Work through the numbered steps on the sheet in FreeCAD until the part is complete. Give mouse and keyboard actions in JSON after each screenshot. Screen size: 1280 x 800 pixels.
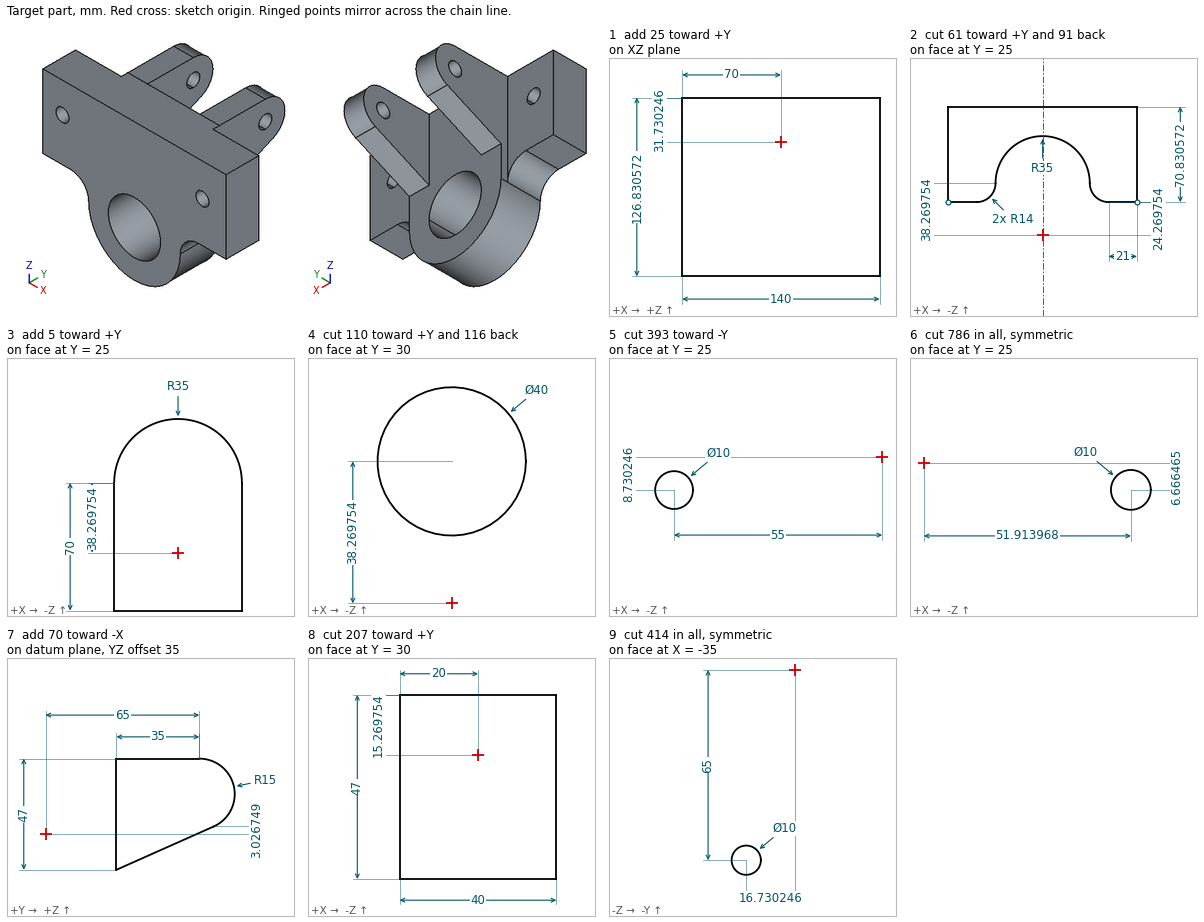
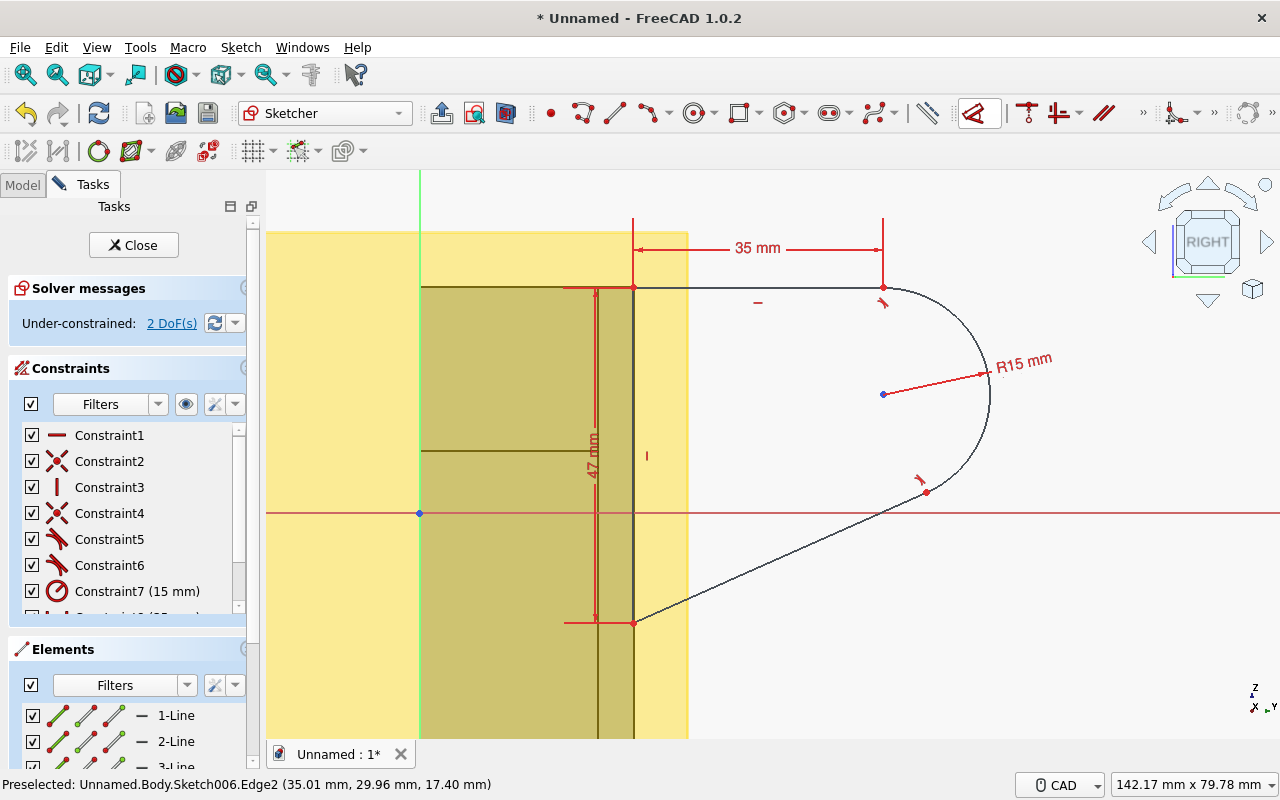
{"action": "left_click", "coordinate": [883, 288]}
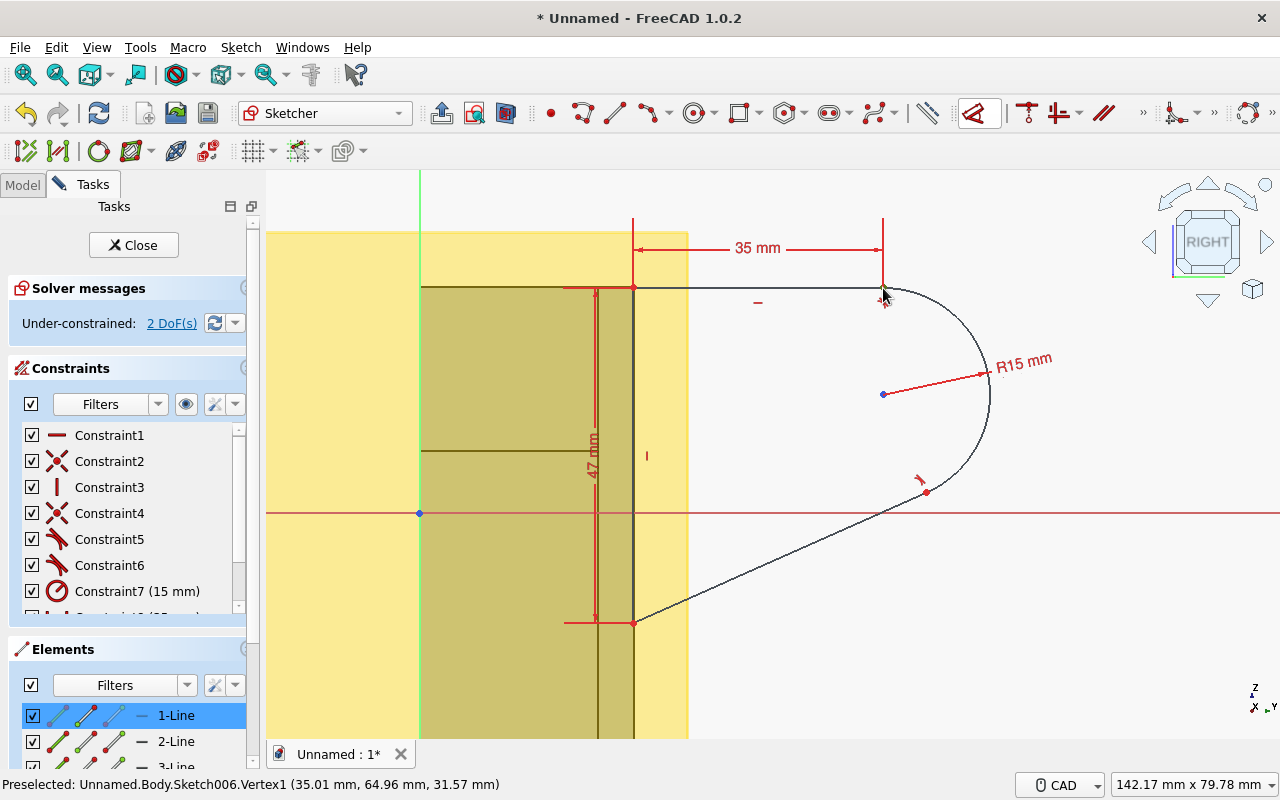
{"action": "left_click", "coordinate": [996, 114]}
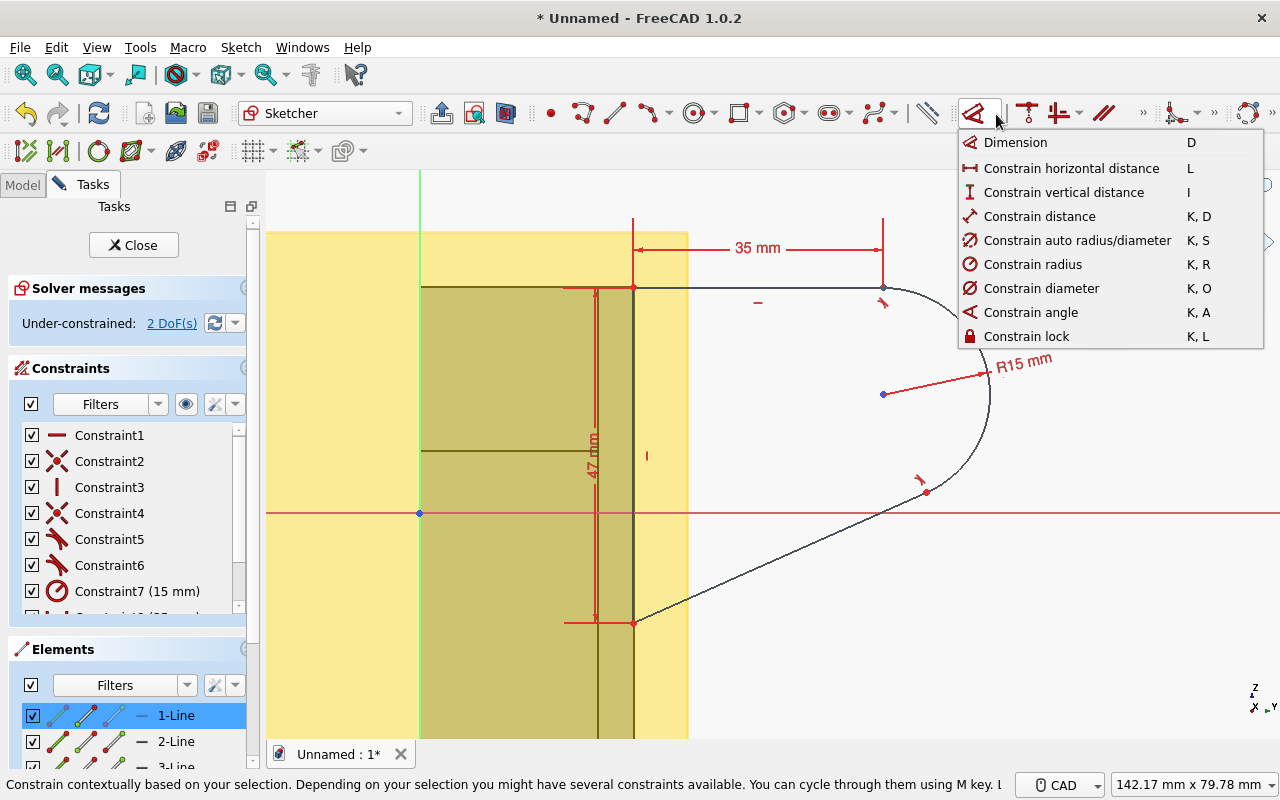
{"action": "left_click", "coordinate": [1111, 168]}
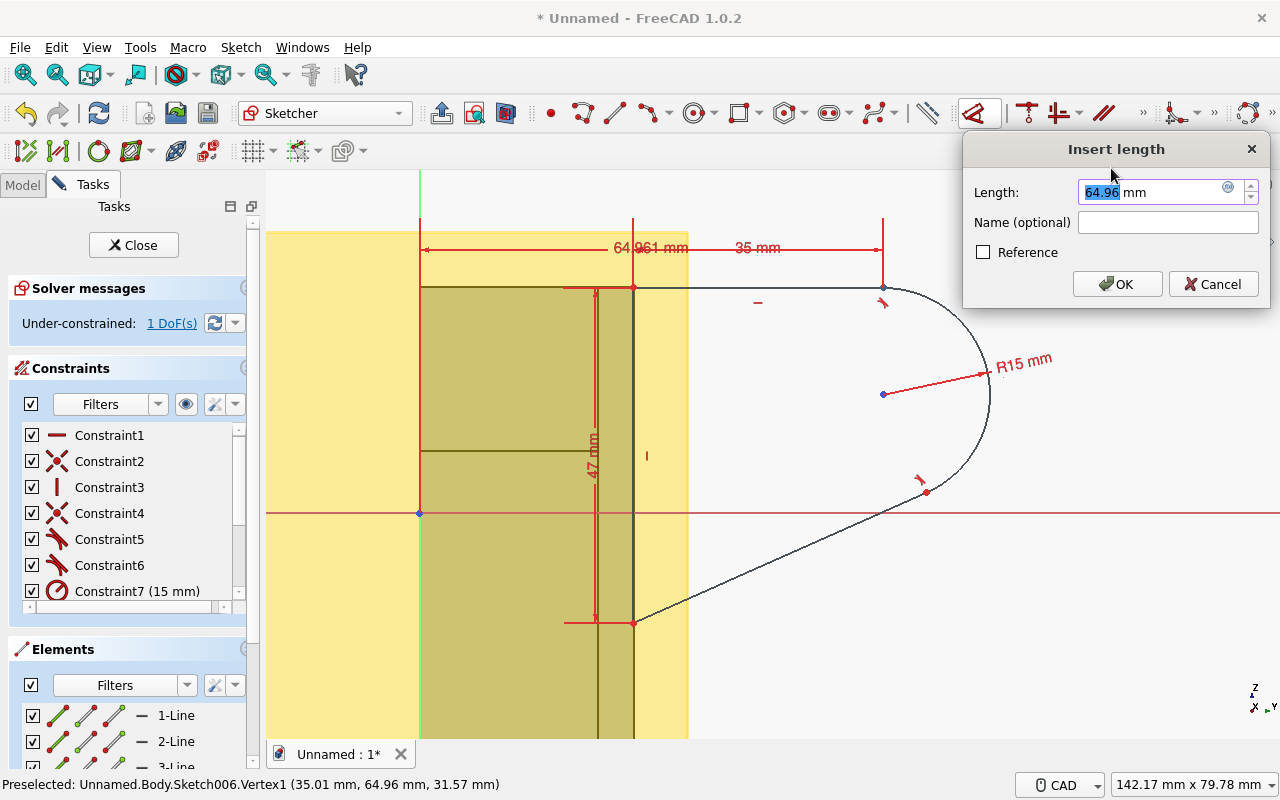
{"action": "type", "text": "65"}
{"action": "key", "text": "Return"}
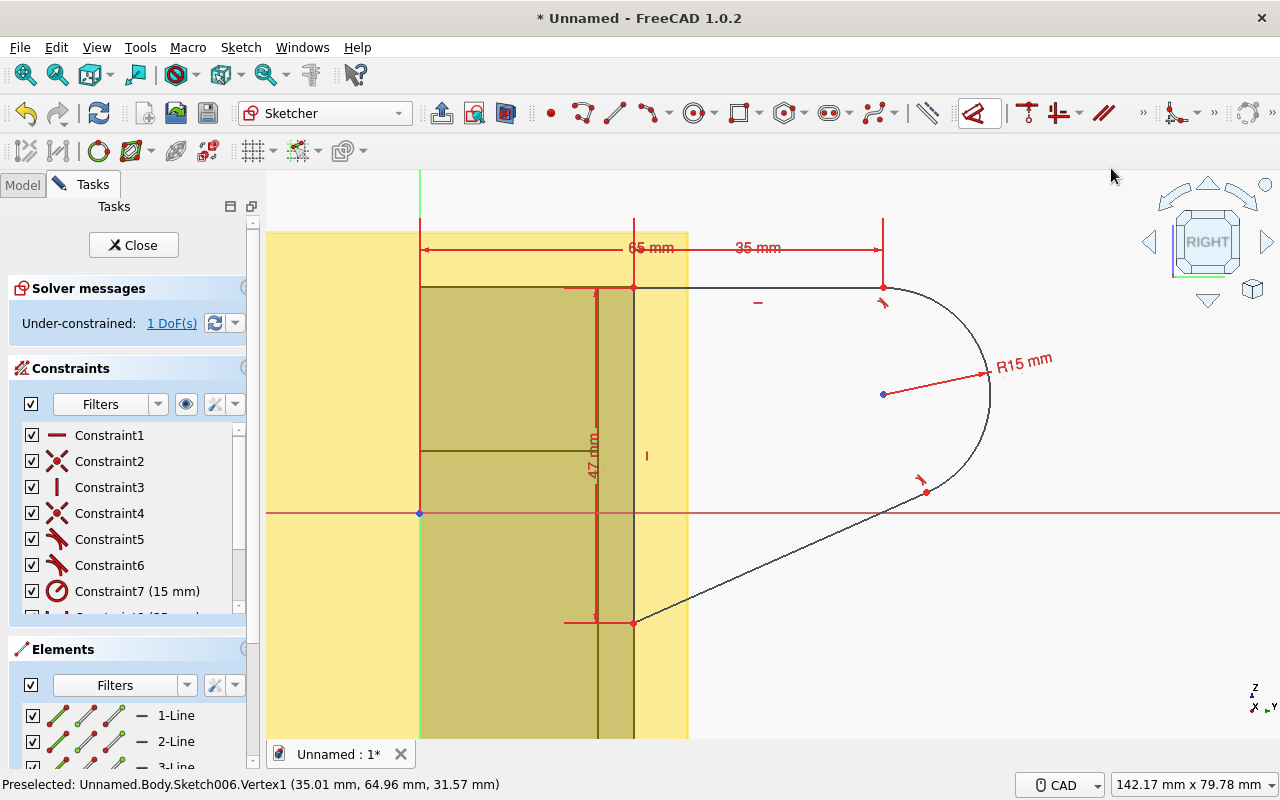
{"action": "scroll", "coordinate": [927, 493], "scroll_direction": "up", "scroll_amount": 4}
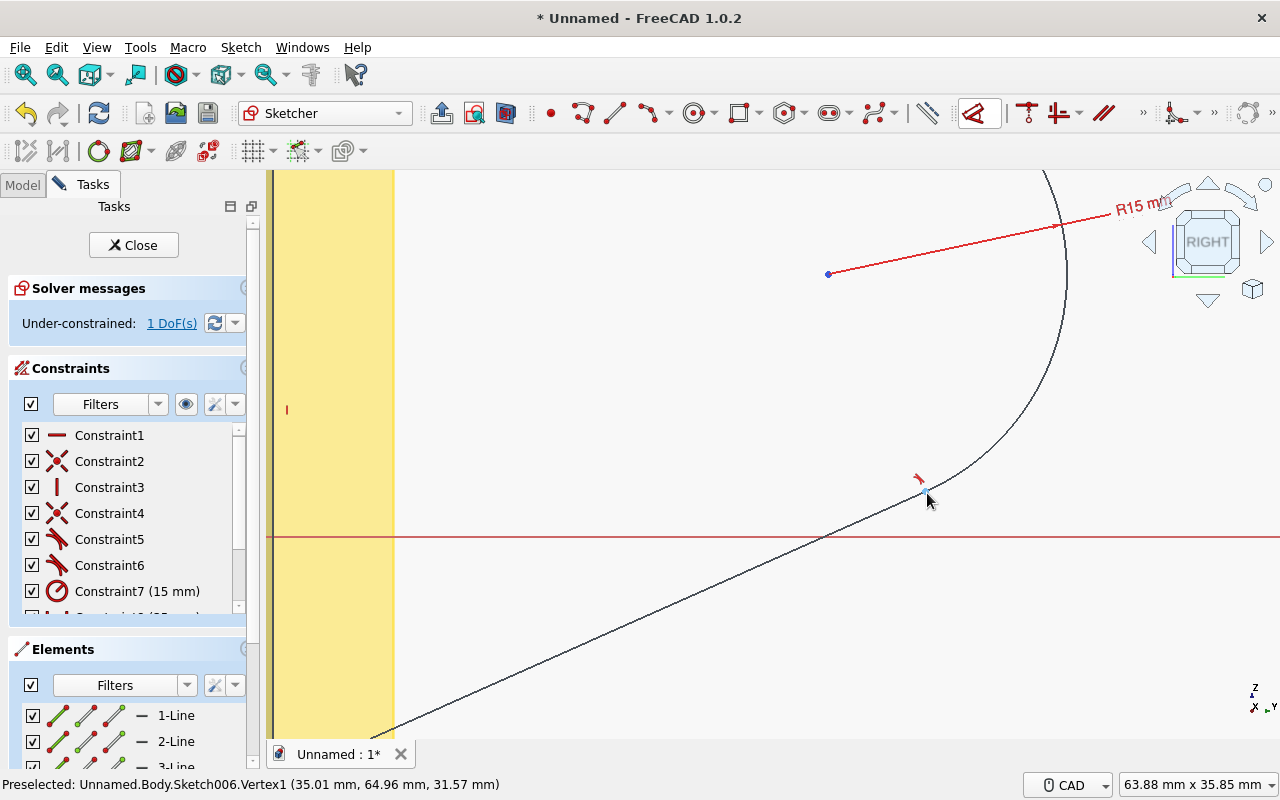
{"action": "left_click", "coordinate": [926, 492]}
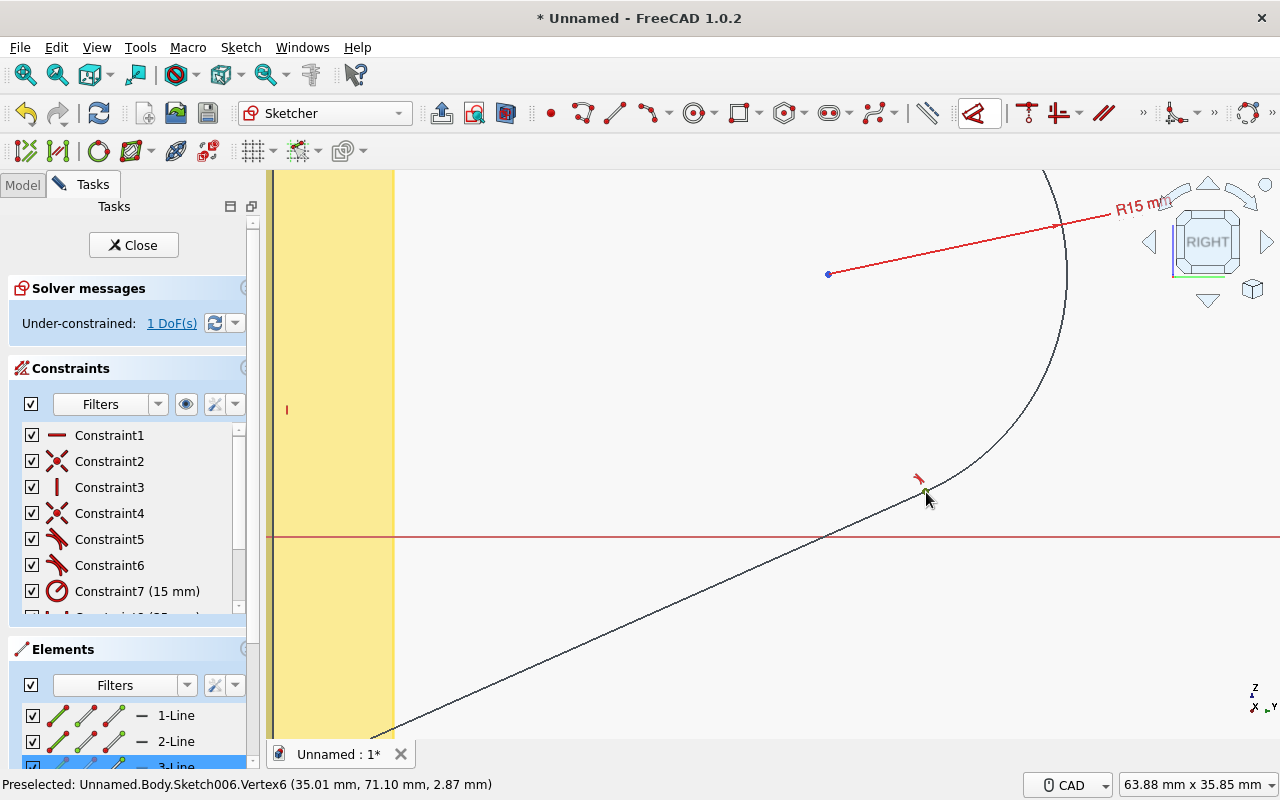
{"action": "left_click", "coordinate": [996, 114]}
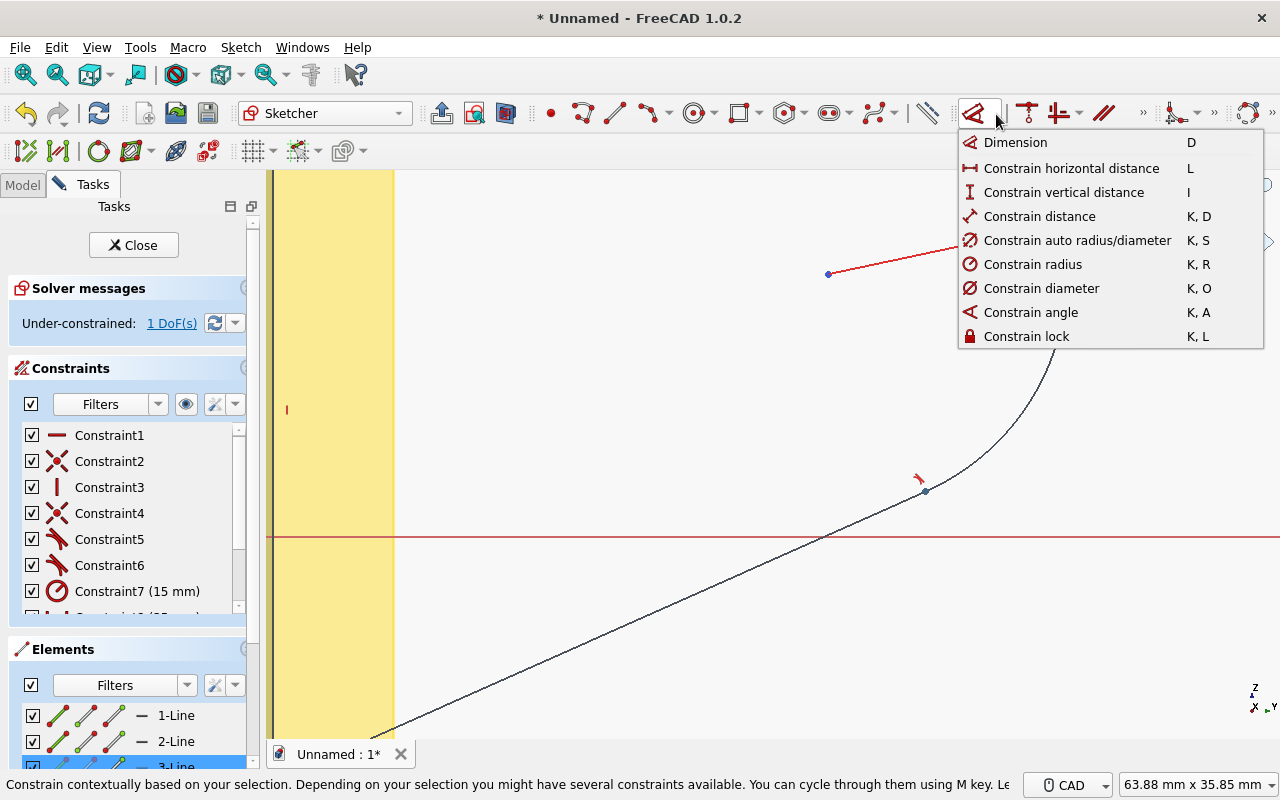
{"action": "left_click", "coordinate": [1111, 192]}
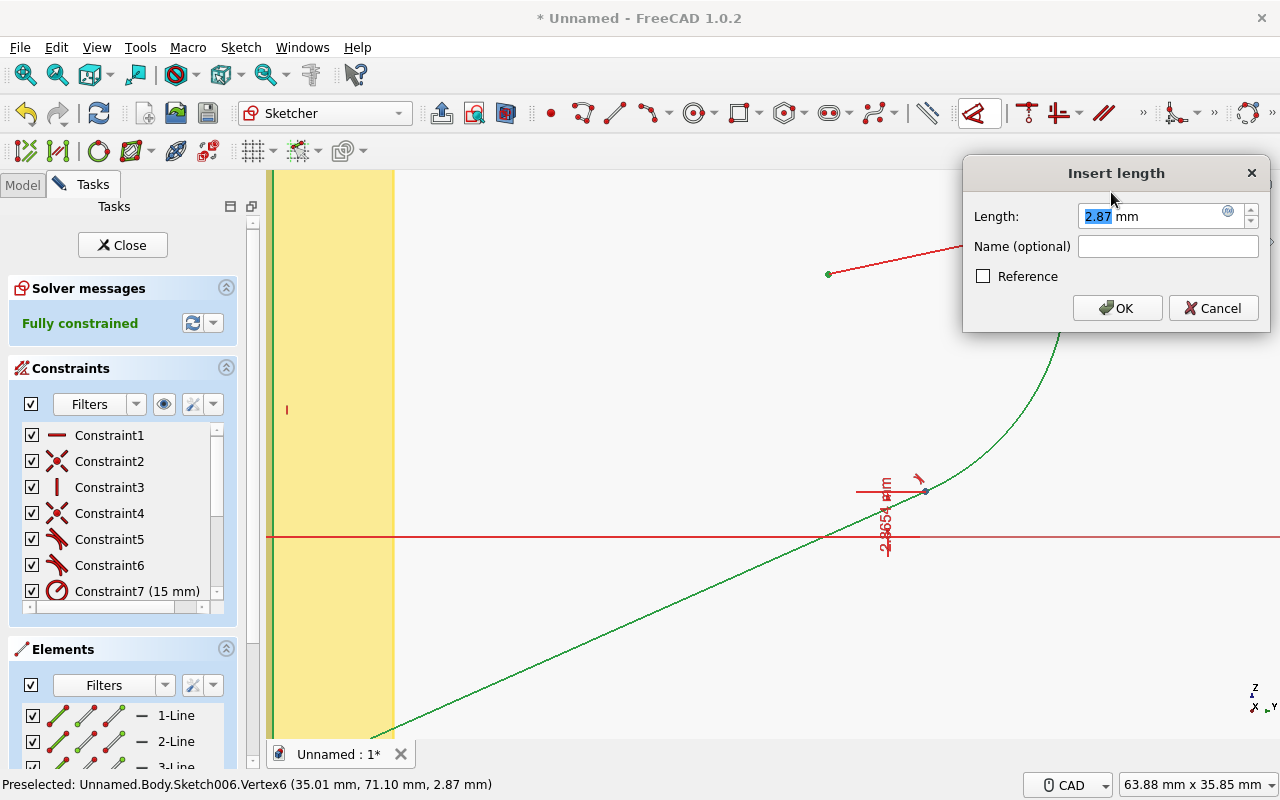
{"action": "type", "text": "3.026749"}
{"action": "key", "text": "Return"}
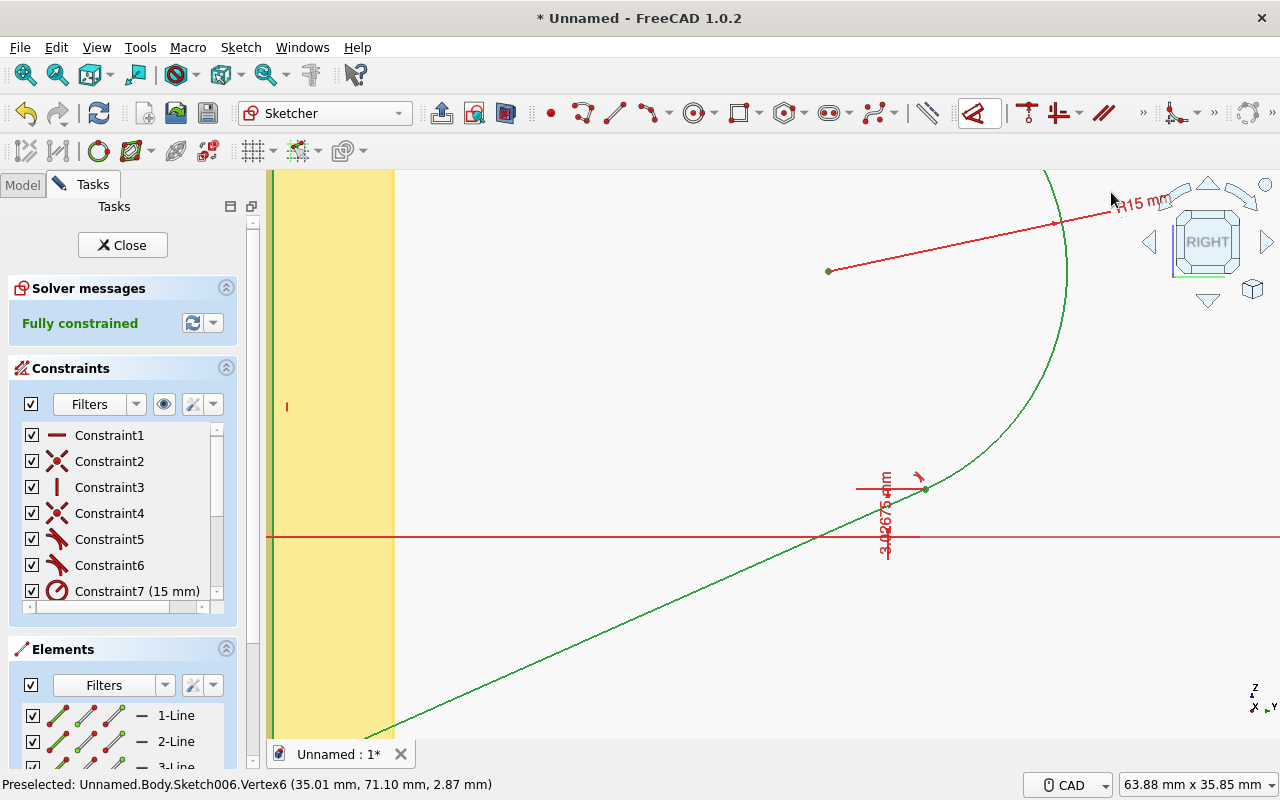
{"action": "left_click", "coordinate": [123, 245]}